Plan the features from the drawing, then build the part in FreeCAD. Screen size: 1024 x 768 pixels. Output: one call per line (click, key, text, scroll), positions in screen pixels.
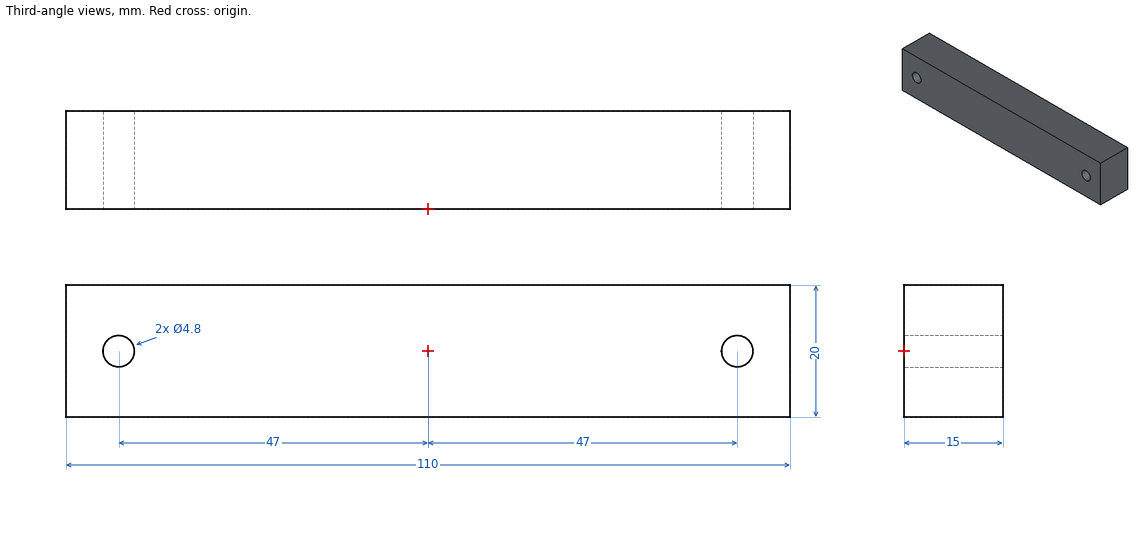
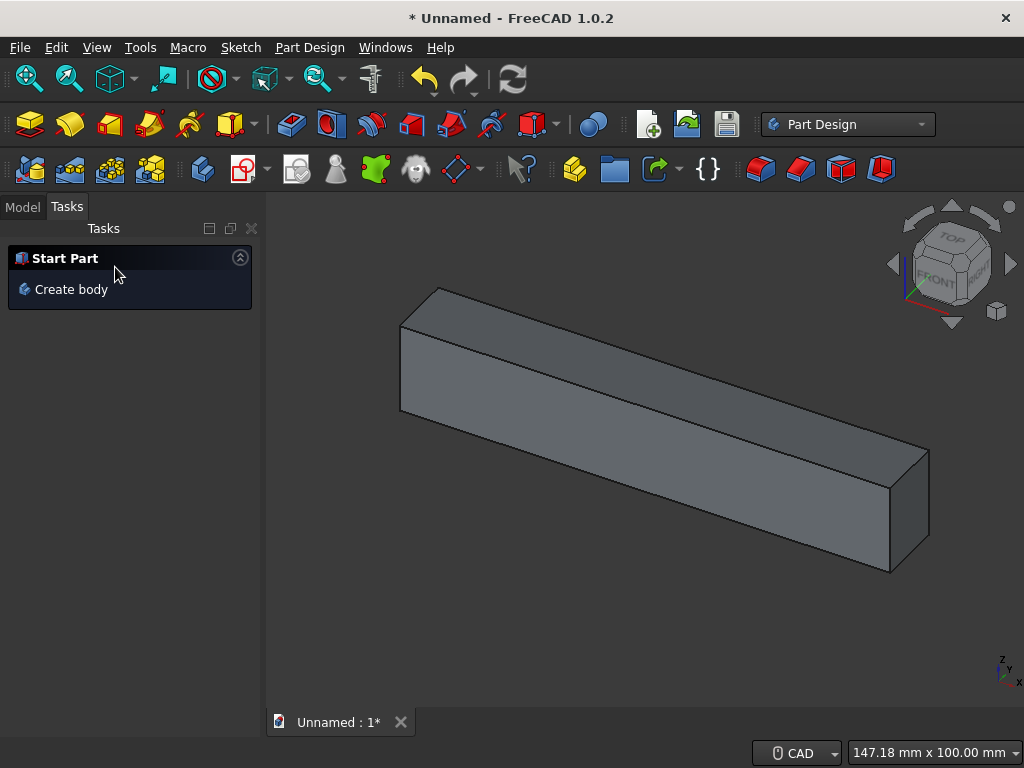
key(4)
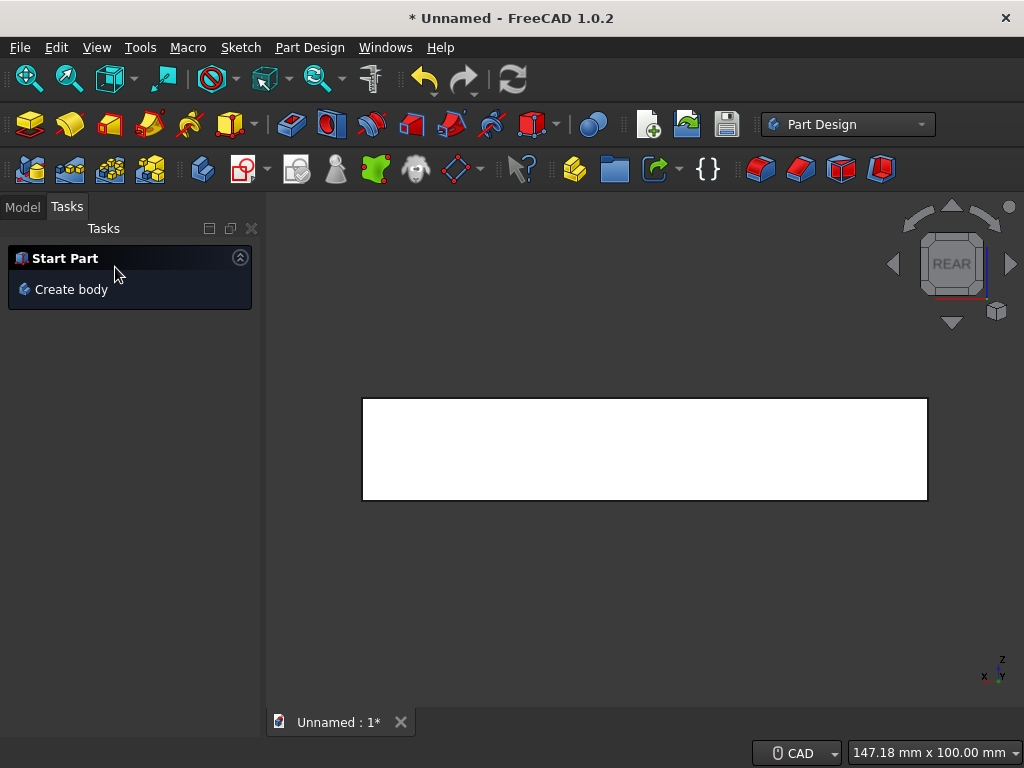
click(483, 448)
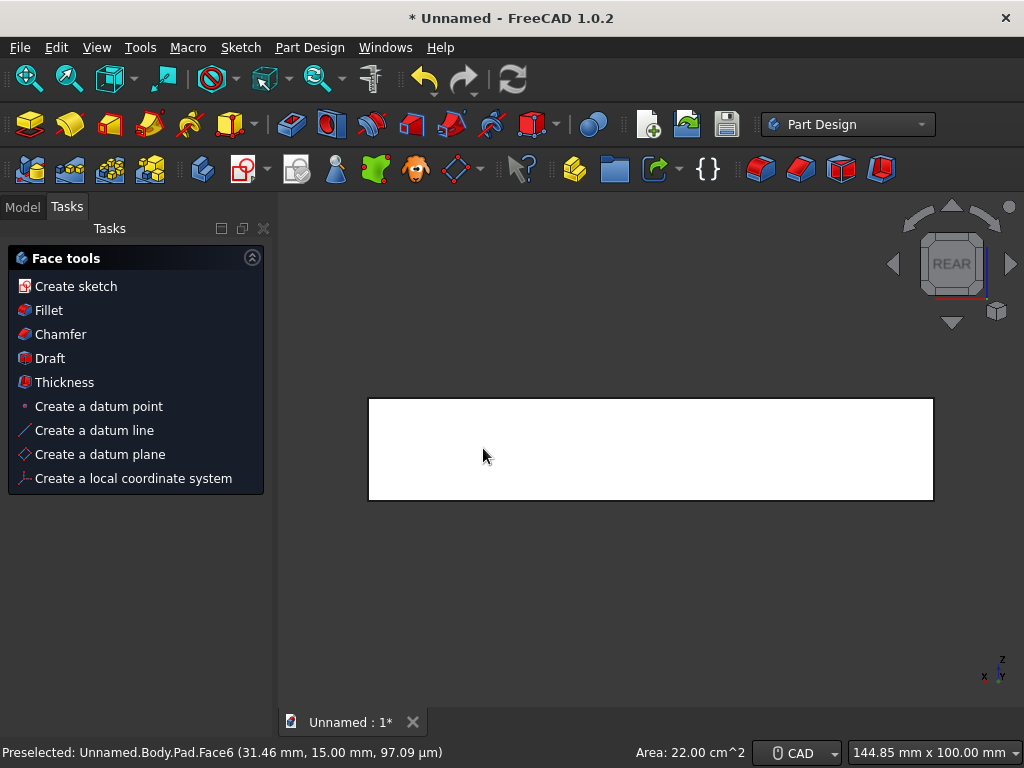
click(244, 170)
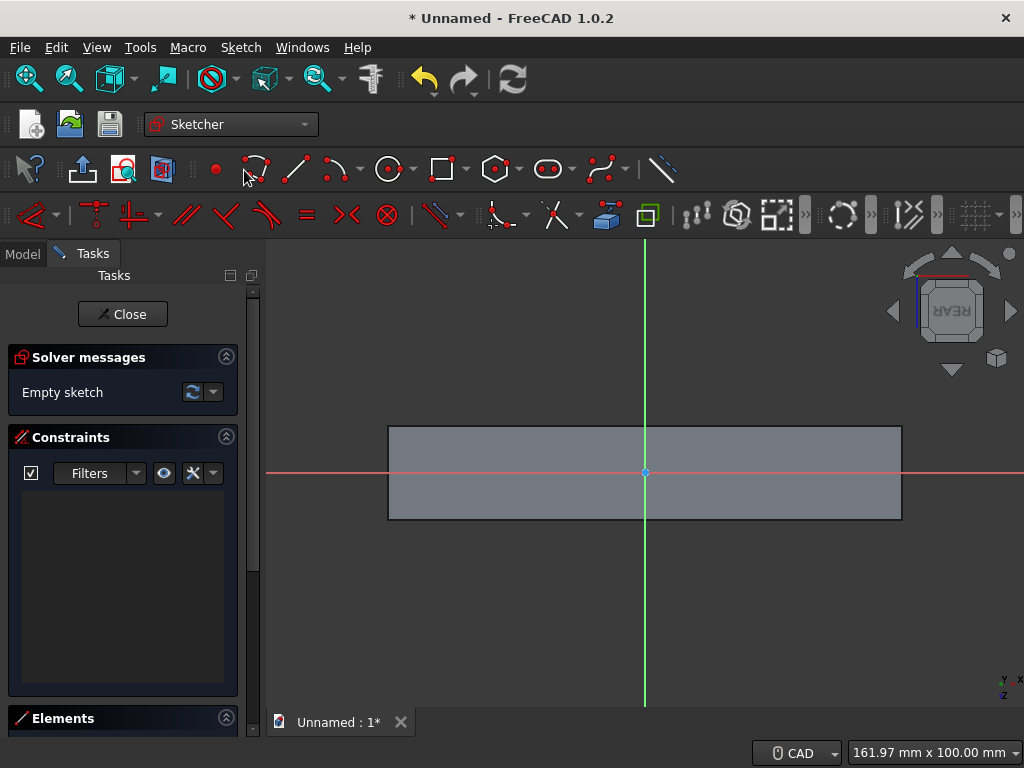
scroll(294, 473, down, 1)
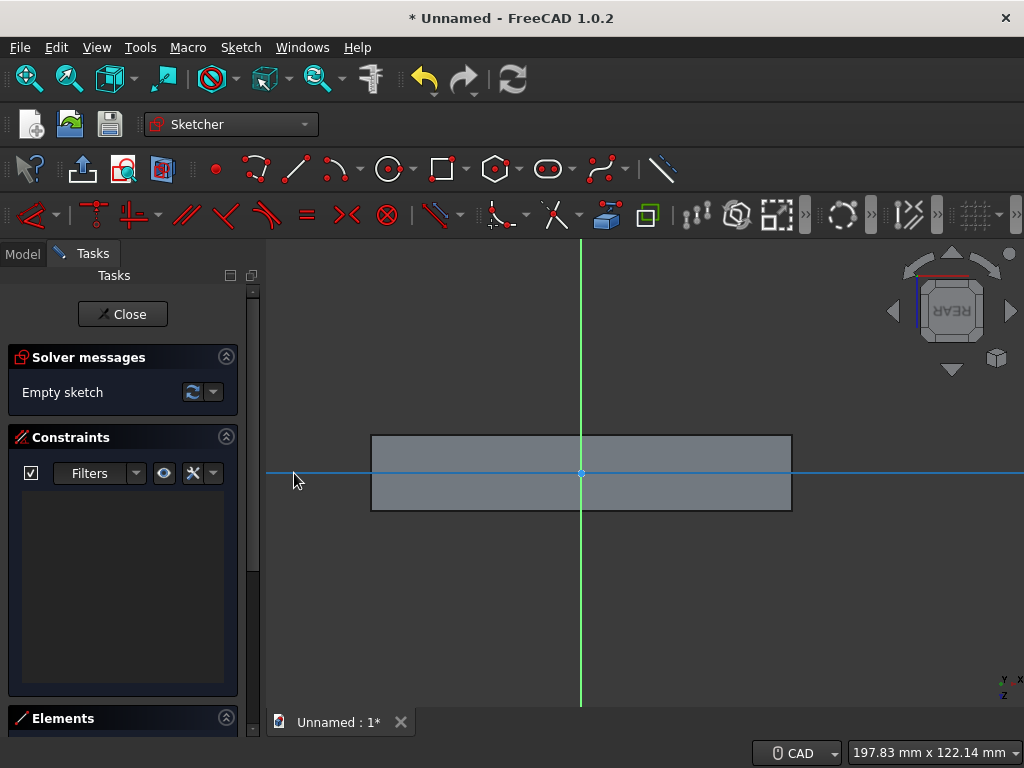
click(390, 170)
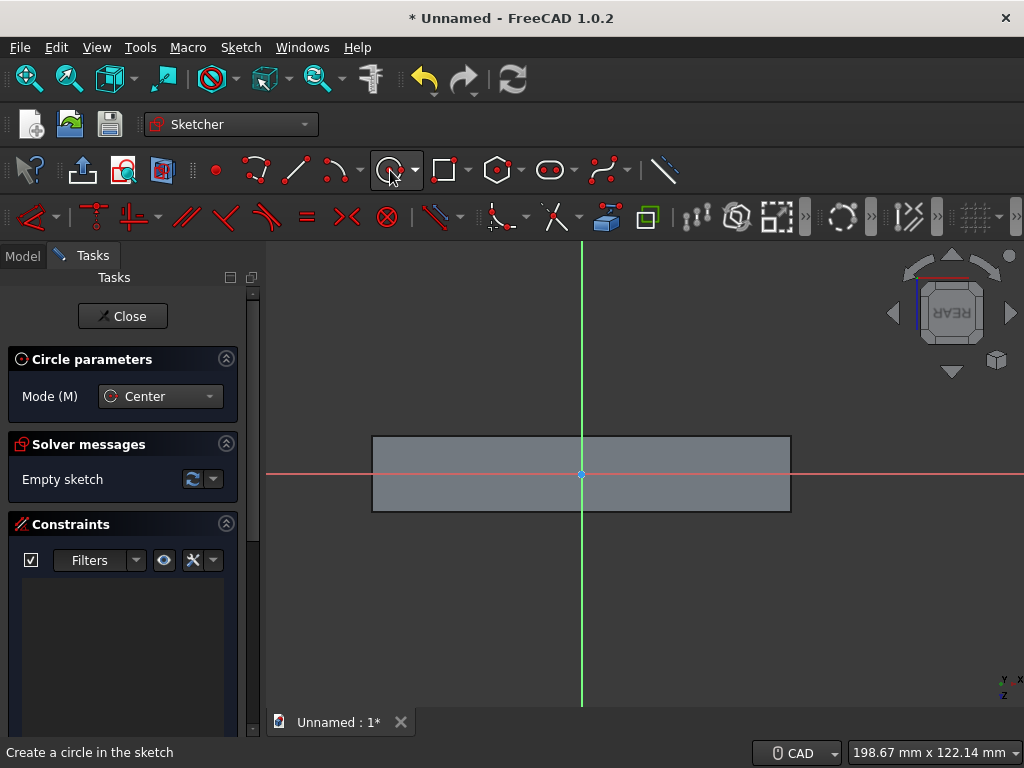
scroll(402, 474, up, 5)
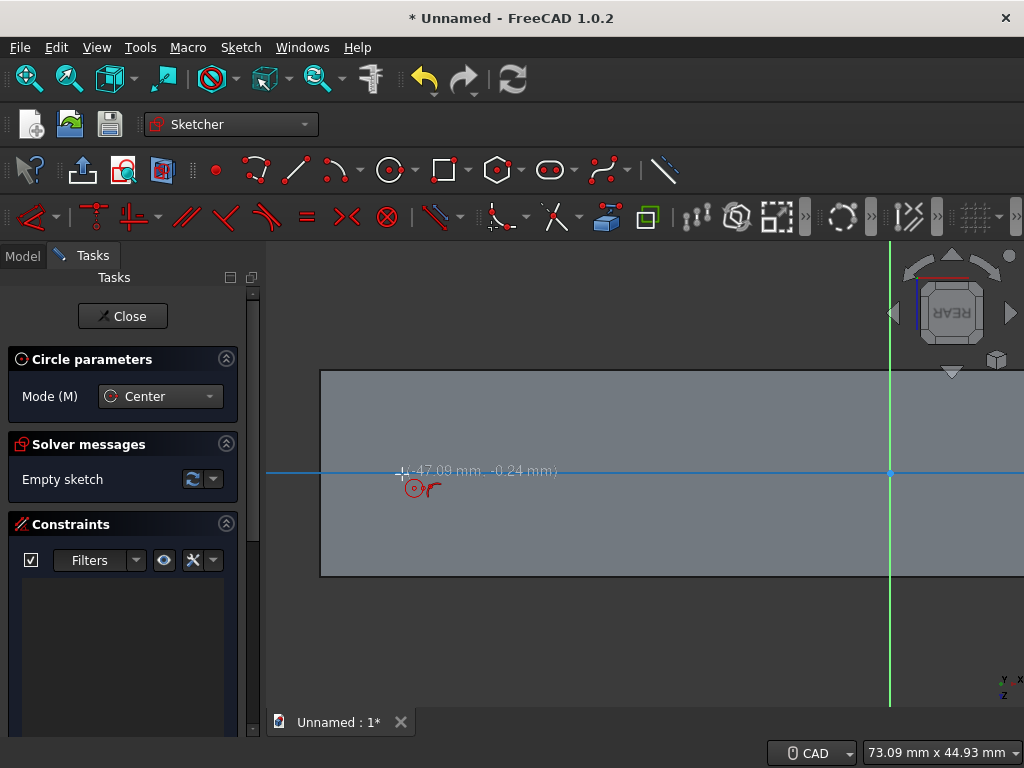
click(403, 473)
move(420, 456)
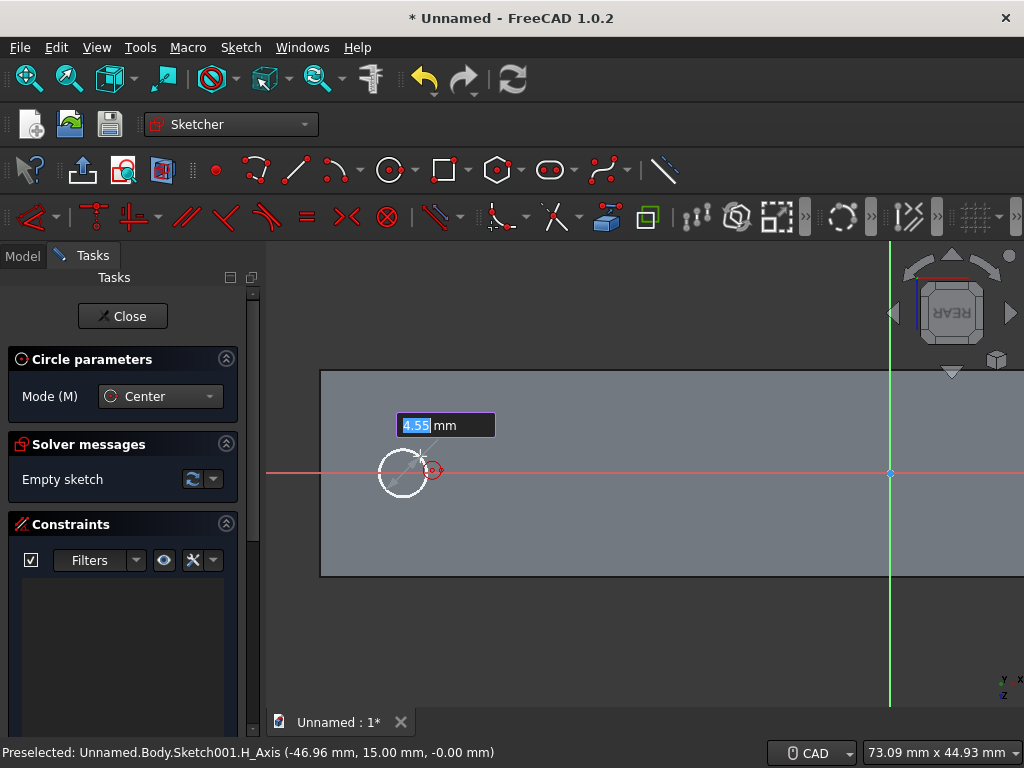
text(4.8)
key(Return)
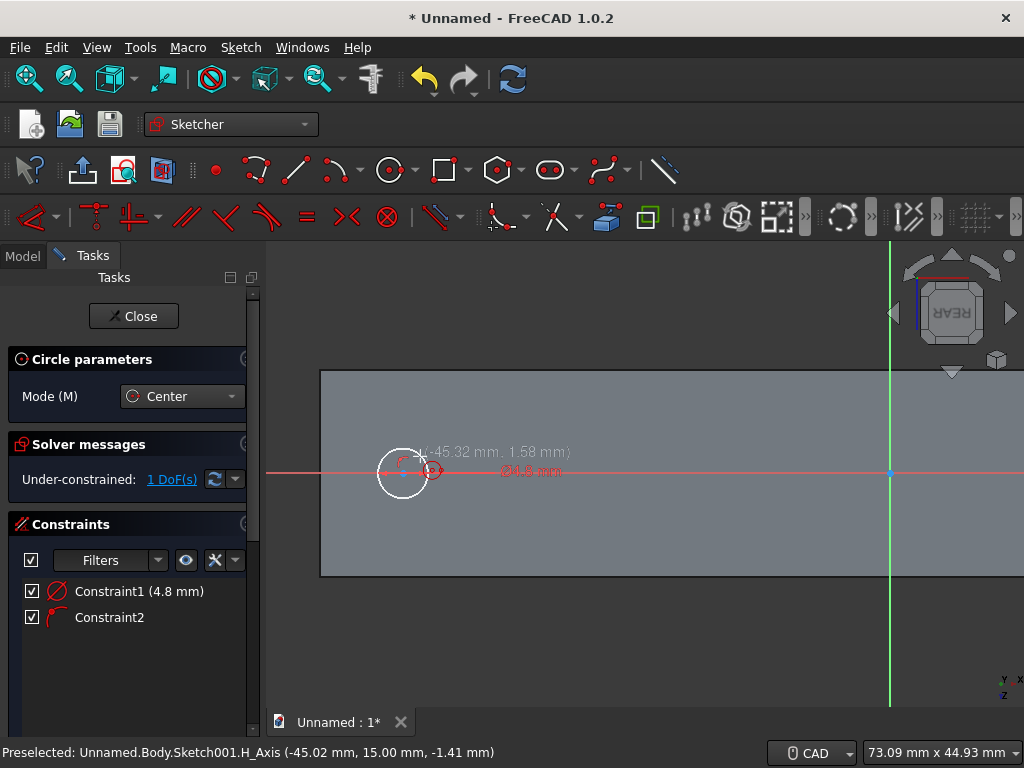
scroll(394, 474, down, 5)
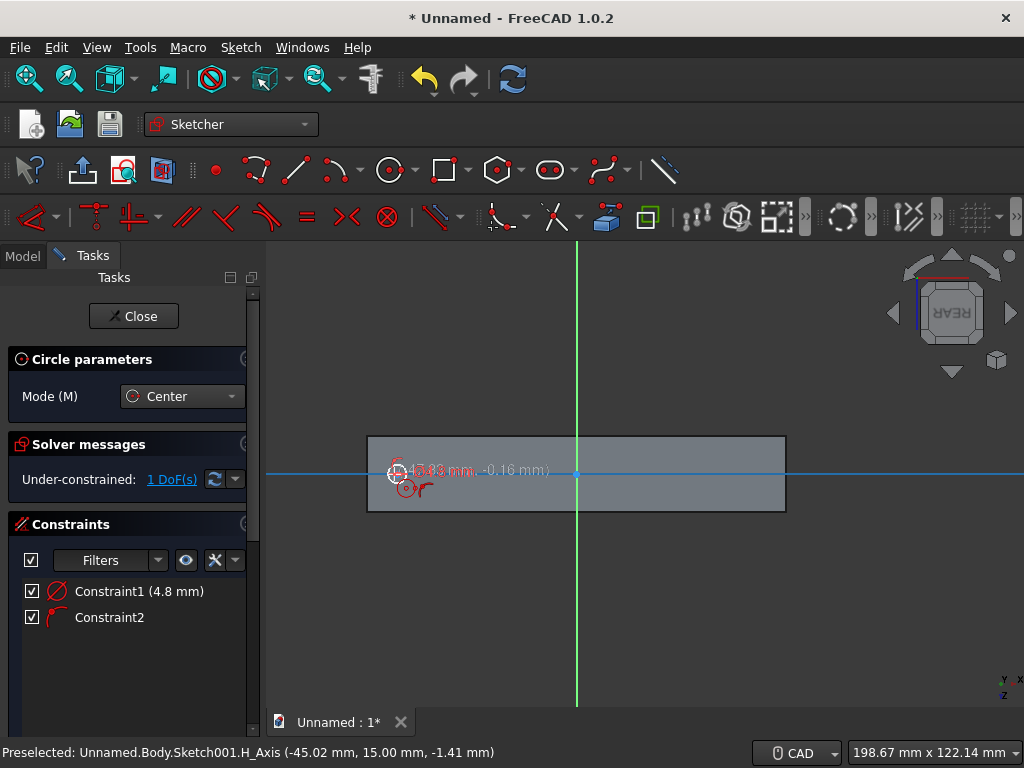
scroll(756, 474, up, 5)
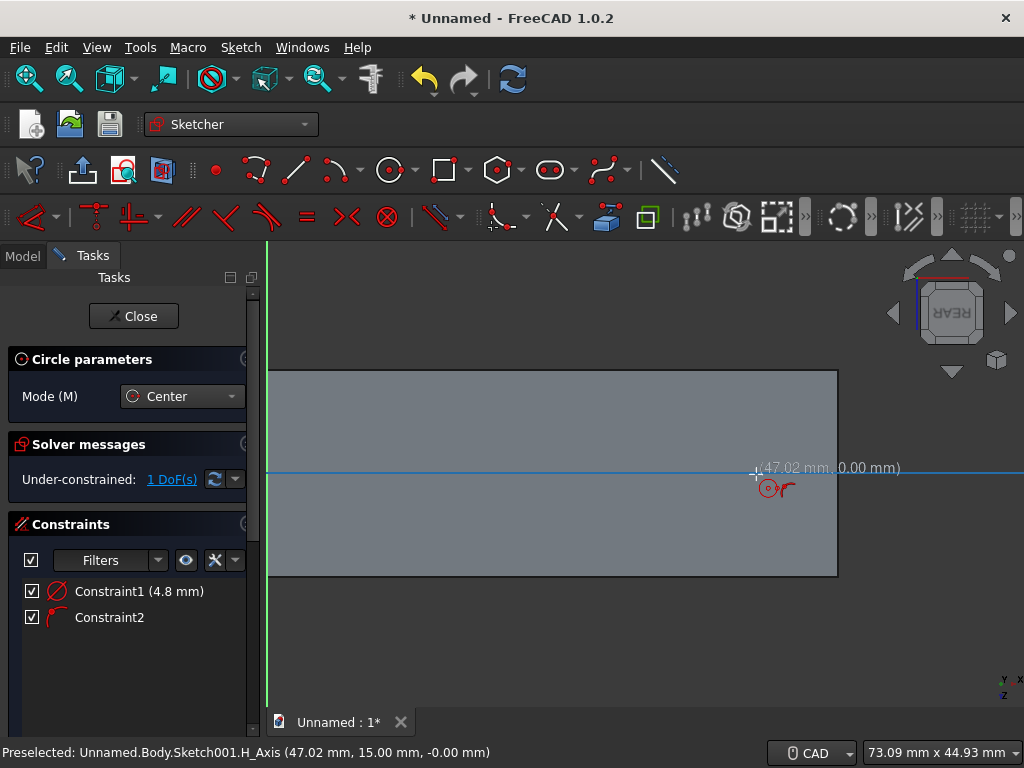
click(755, 473)
move(772, 456)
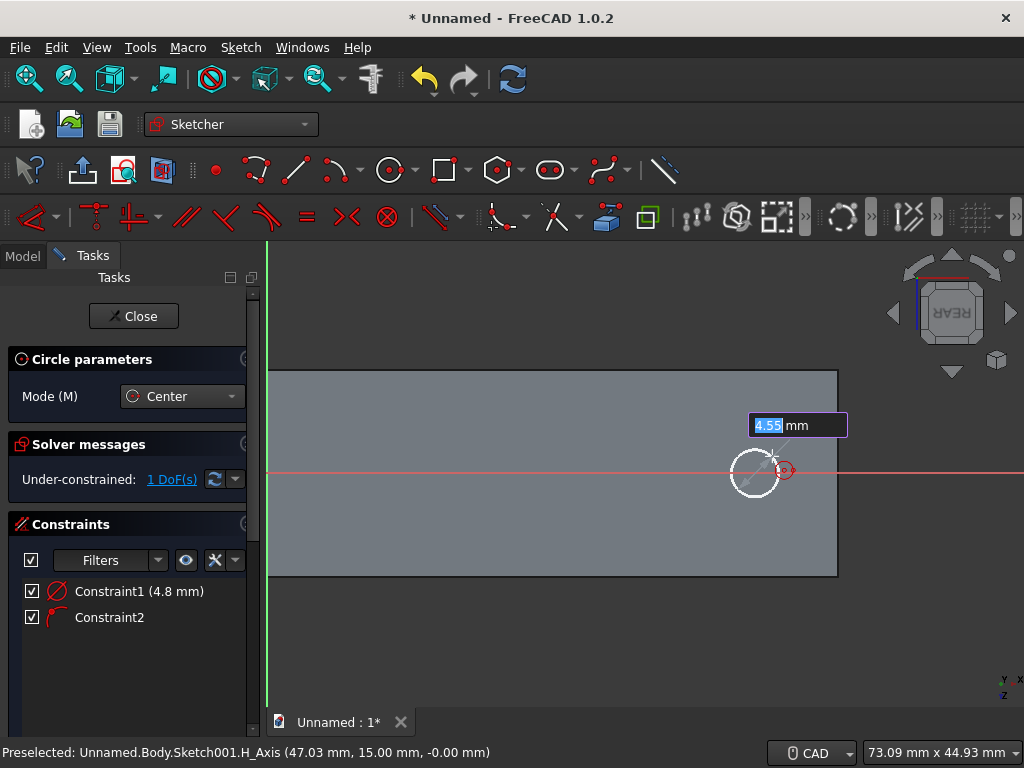
text(4.8)
key(Return)
key(Escape)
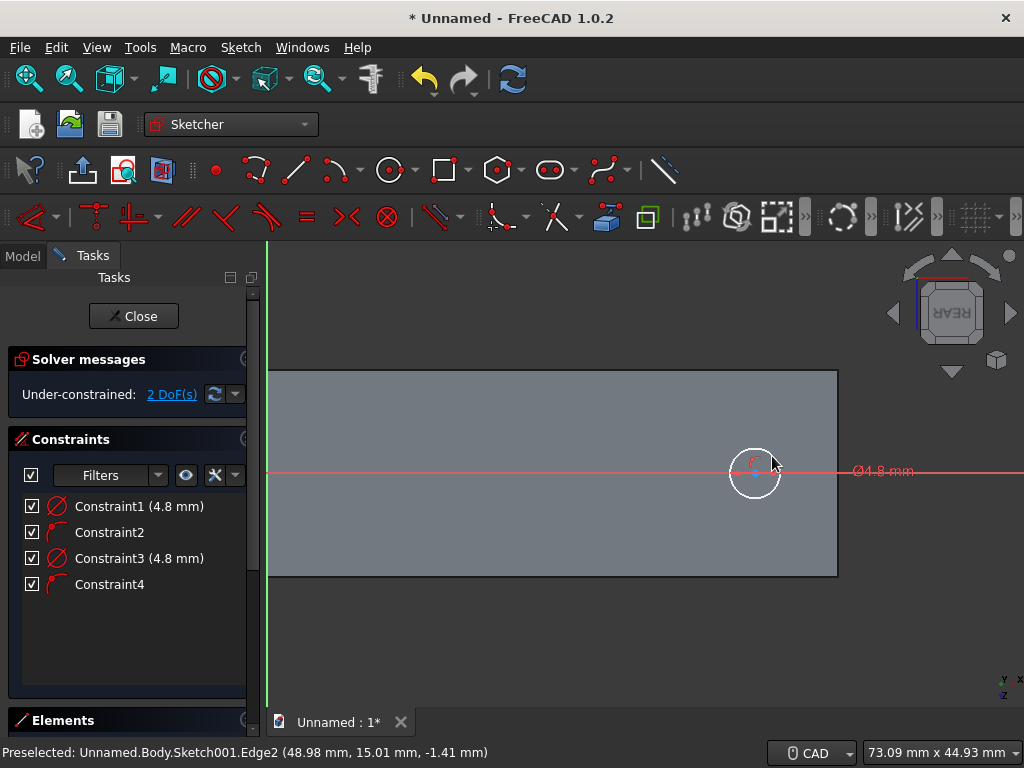
click(32, 218)